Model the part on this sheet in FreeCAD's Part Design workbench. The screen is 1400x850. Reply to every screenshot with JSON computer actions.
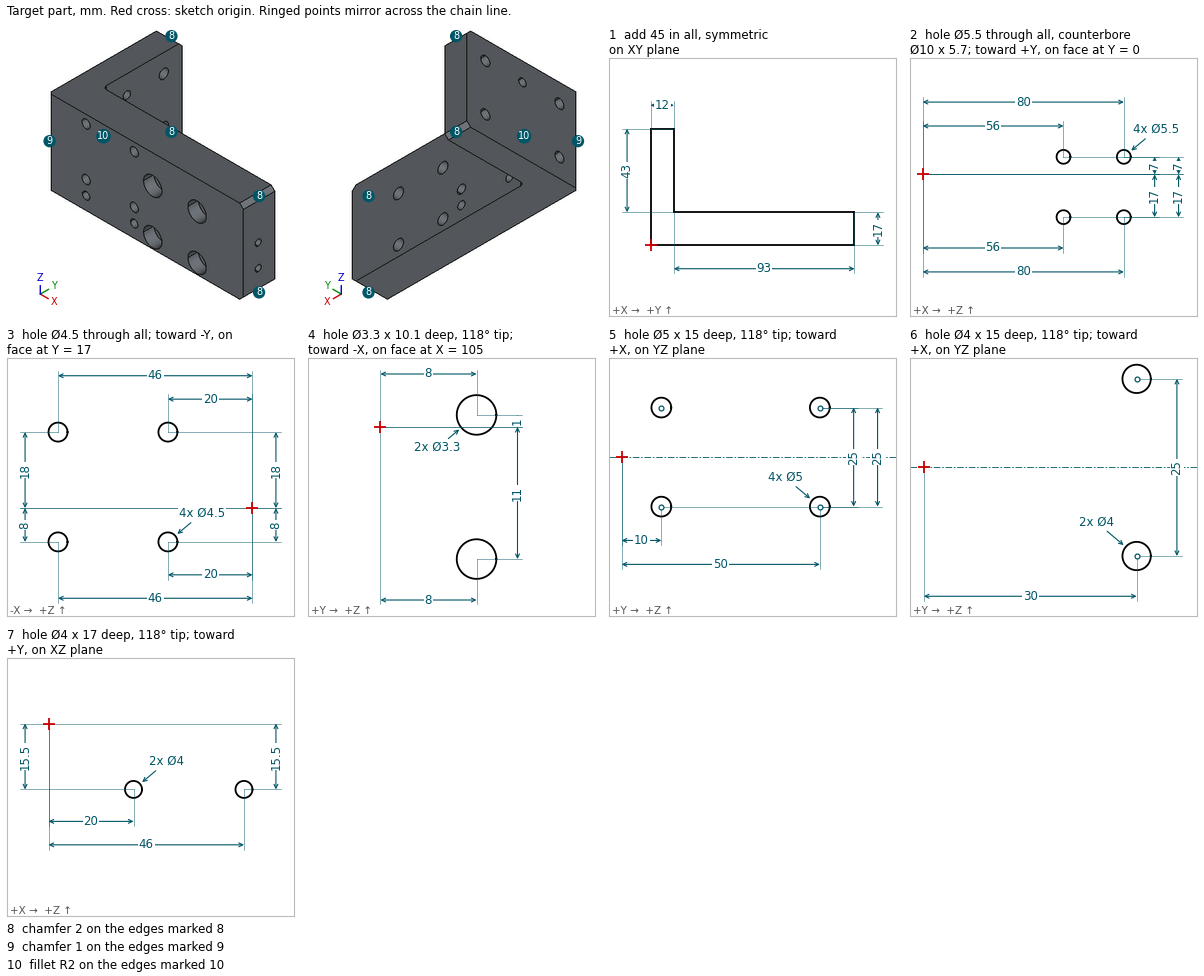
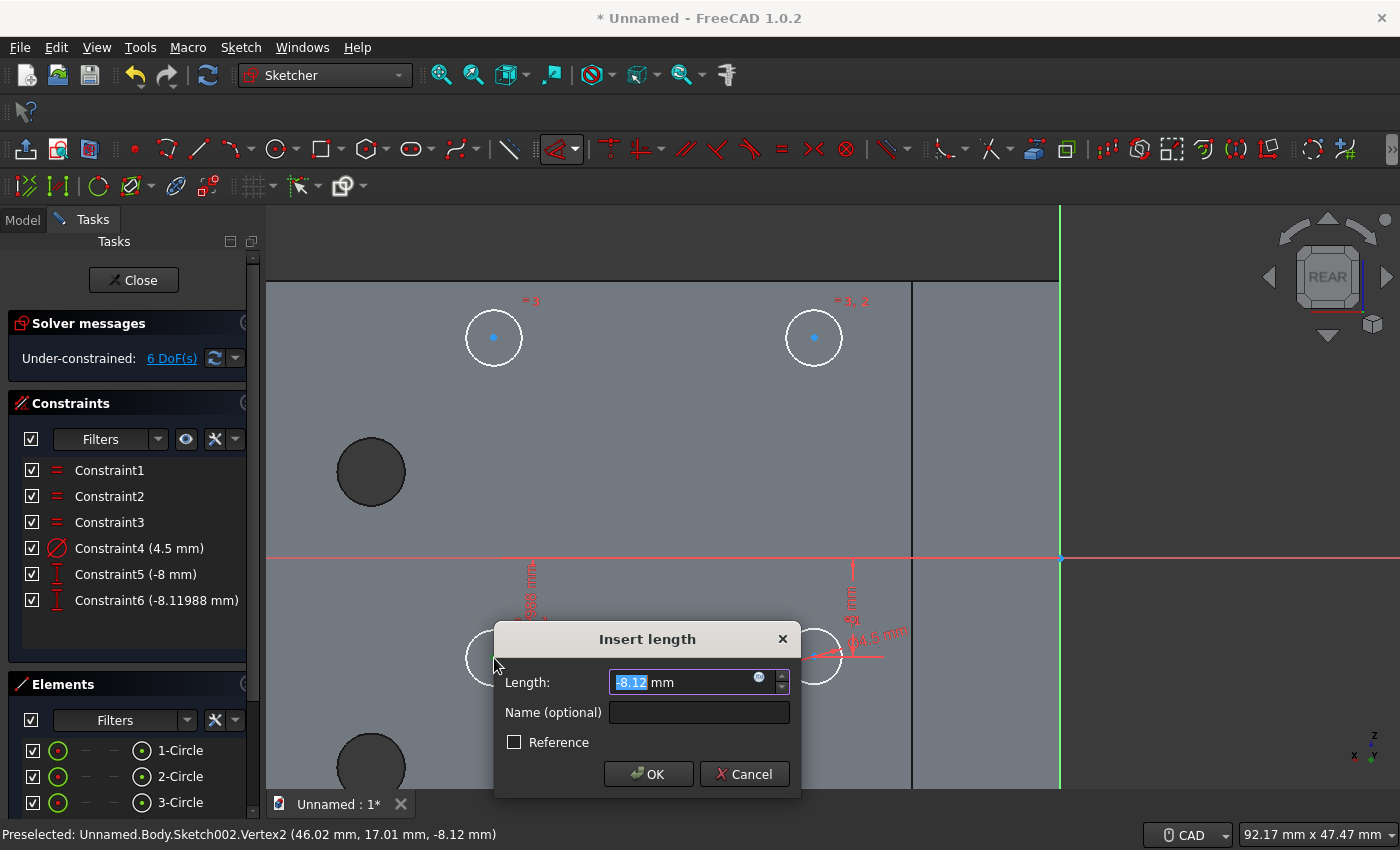
{"action": "type", "text": "-8"}
{"action": "key", "text": "Return"}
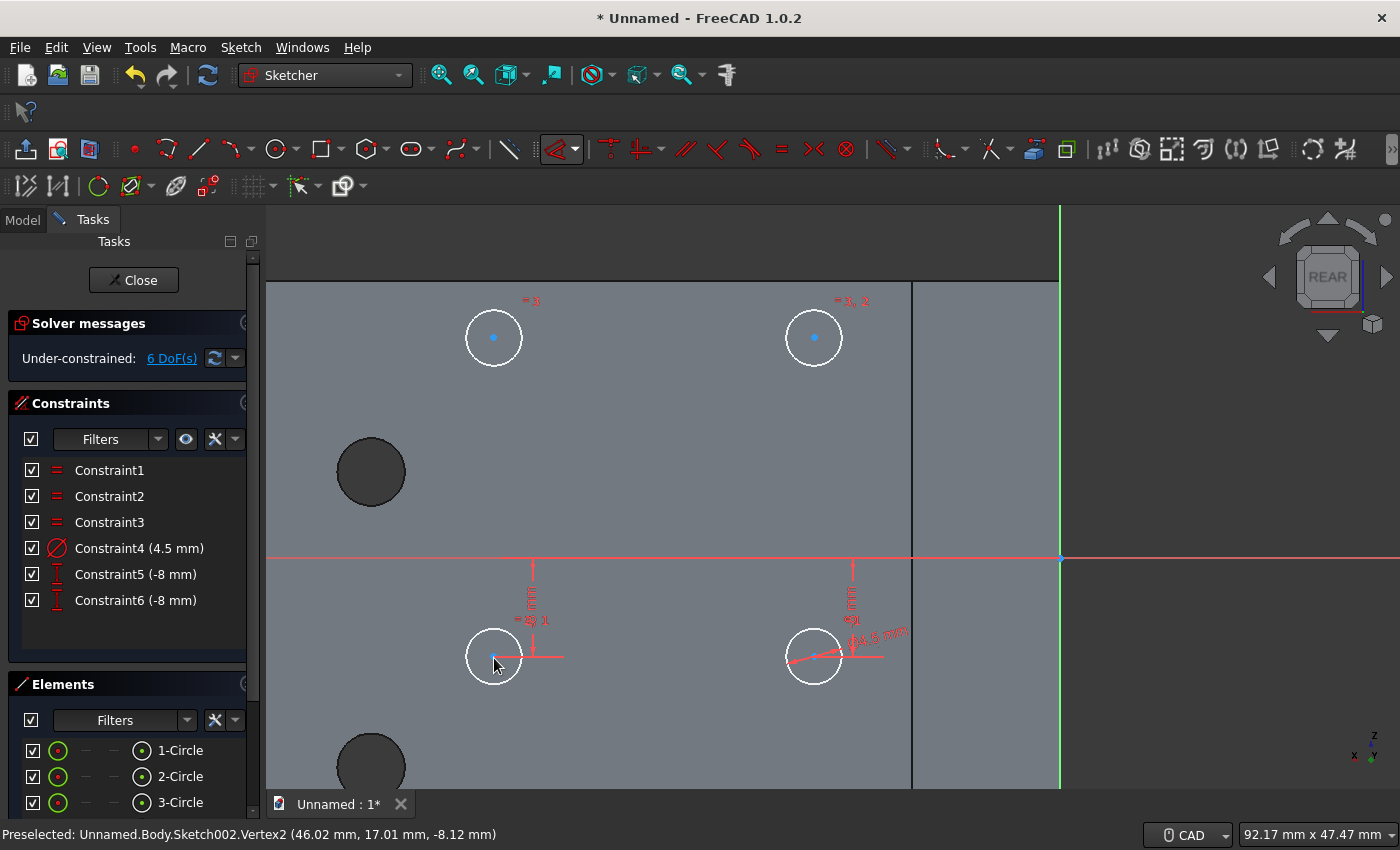
{"action": "left_click", "coordinate": [814, 657]}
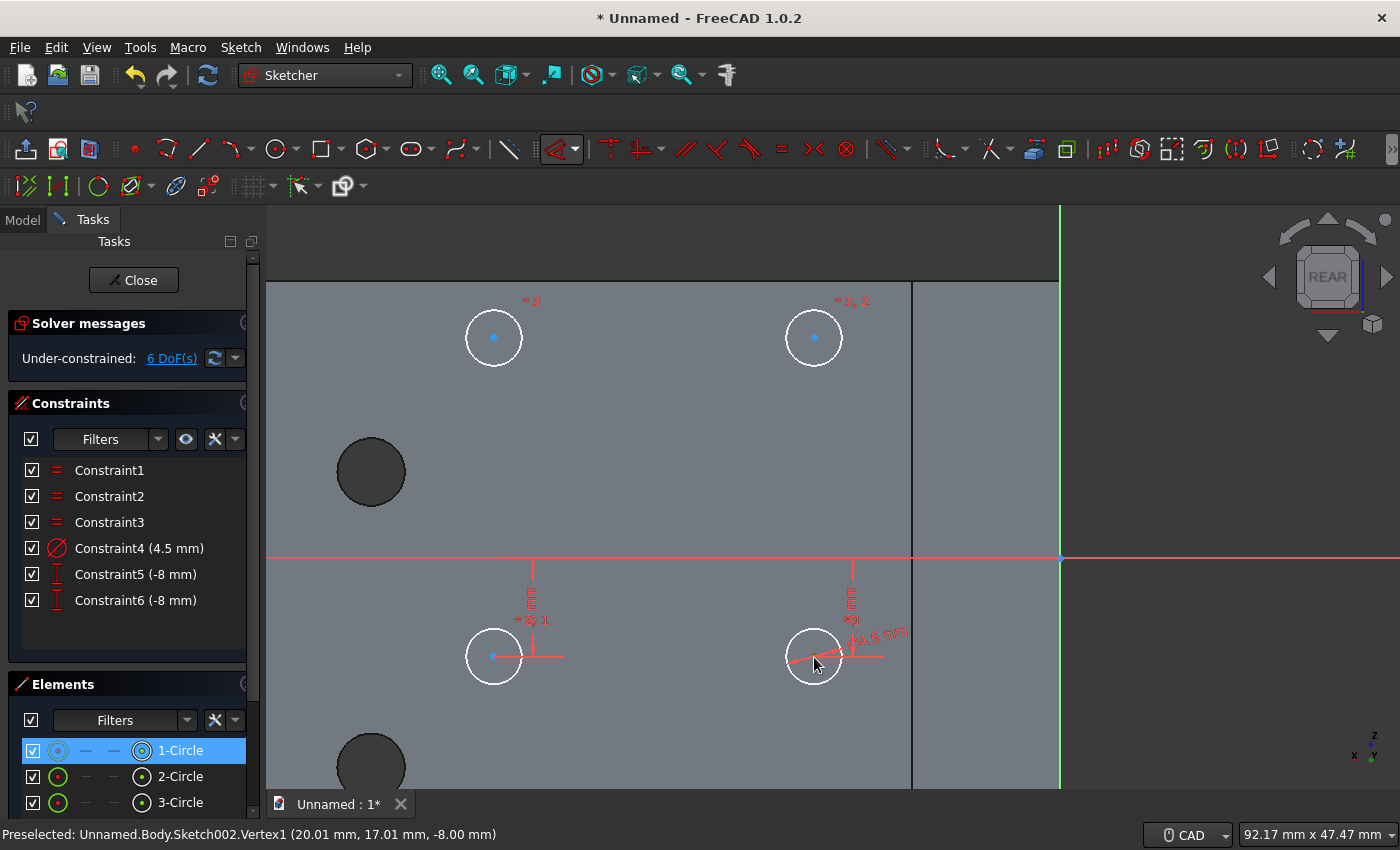
{"action": "key", "text": "l"}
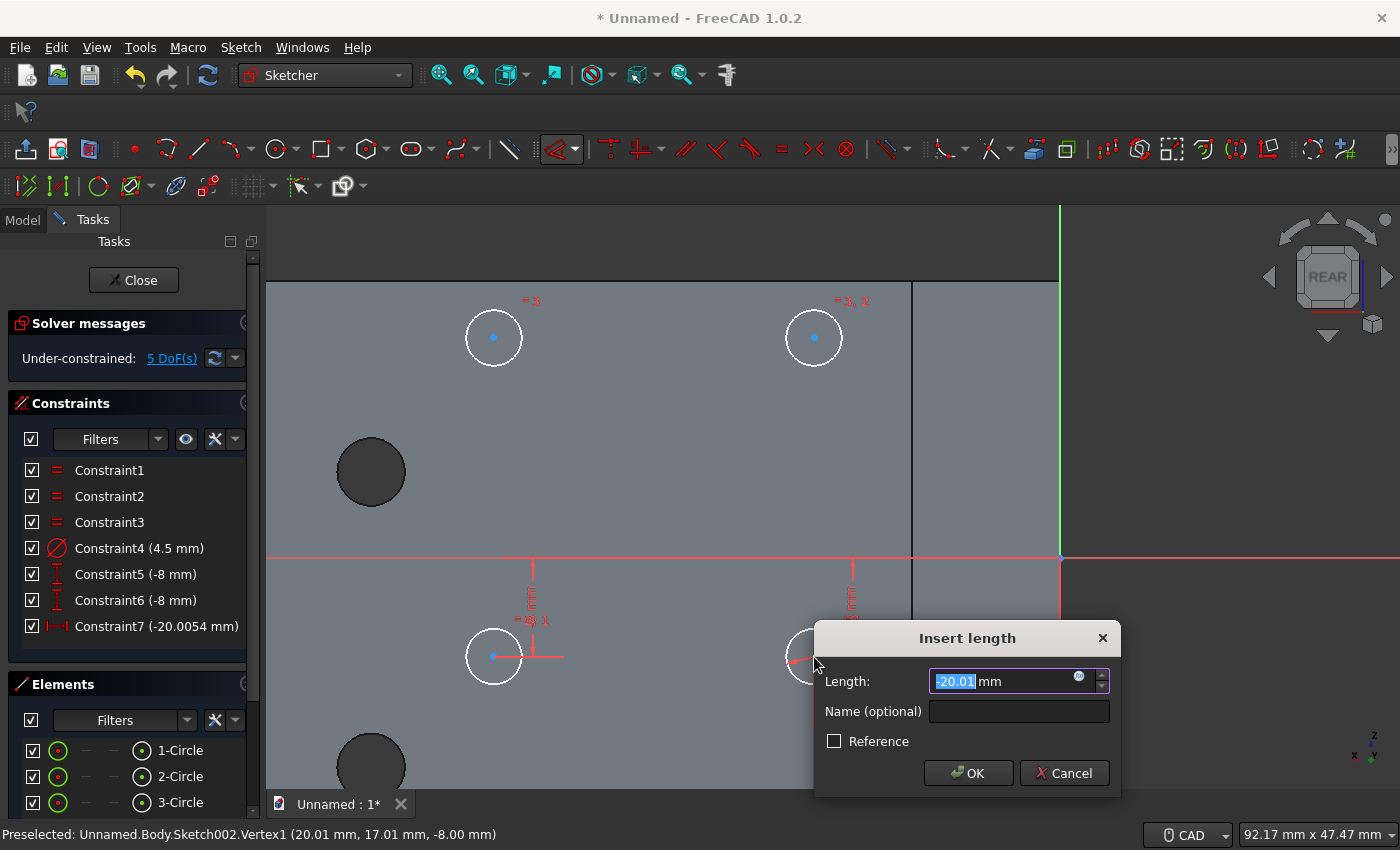
{"action": "type", "text": "-20"}
{"action": "key", "text": "Return"}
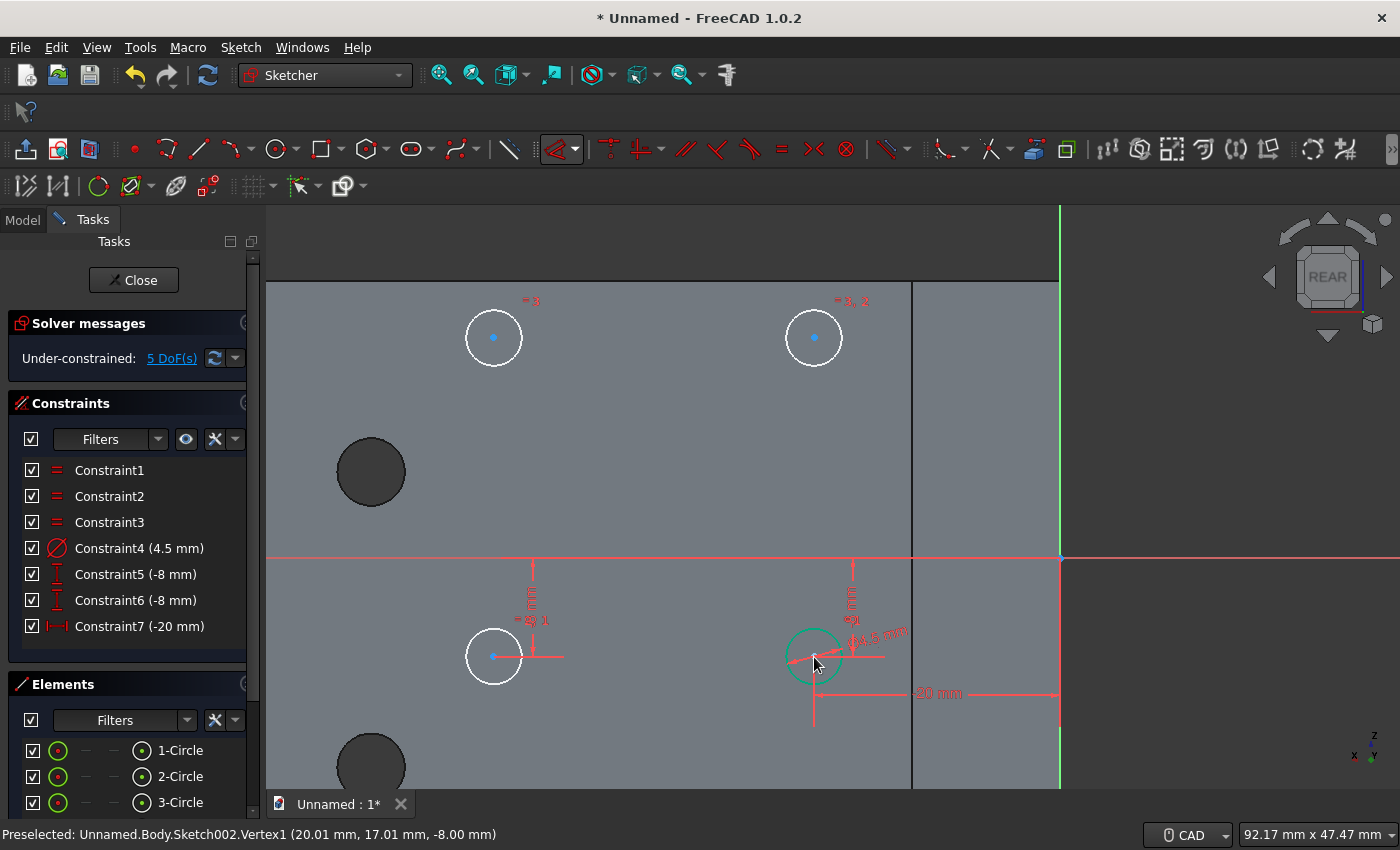
{"action": "left_click", "coordinate": [494, 657]}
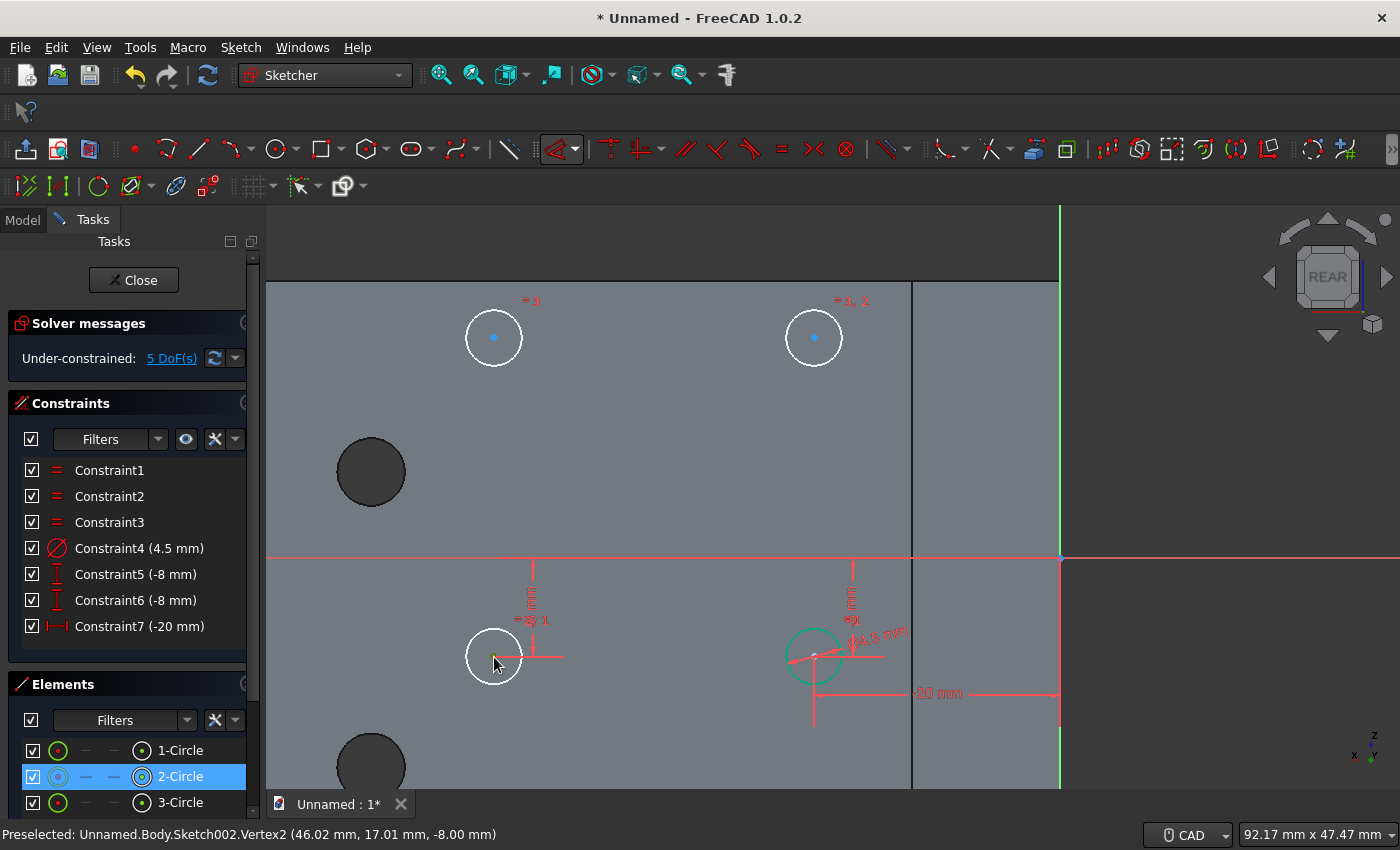
{"action": "key", "text": "l"}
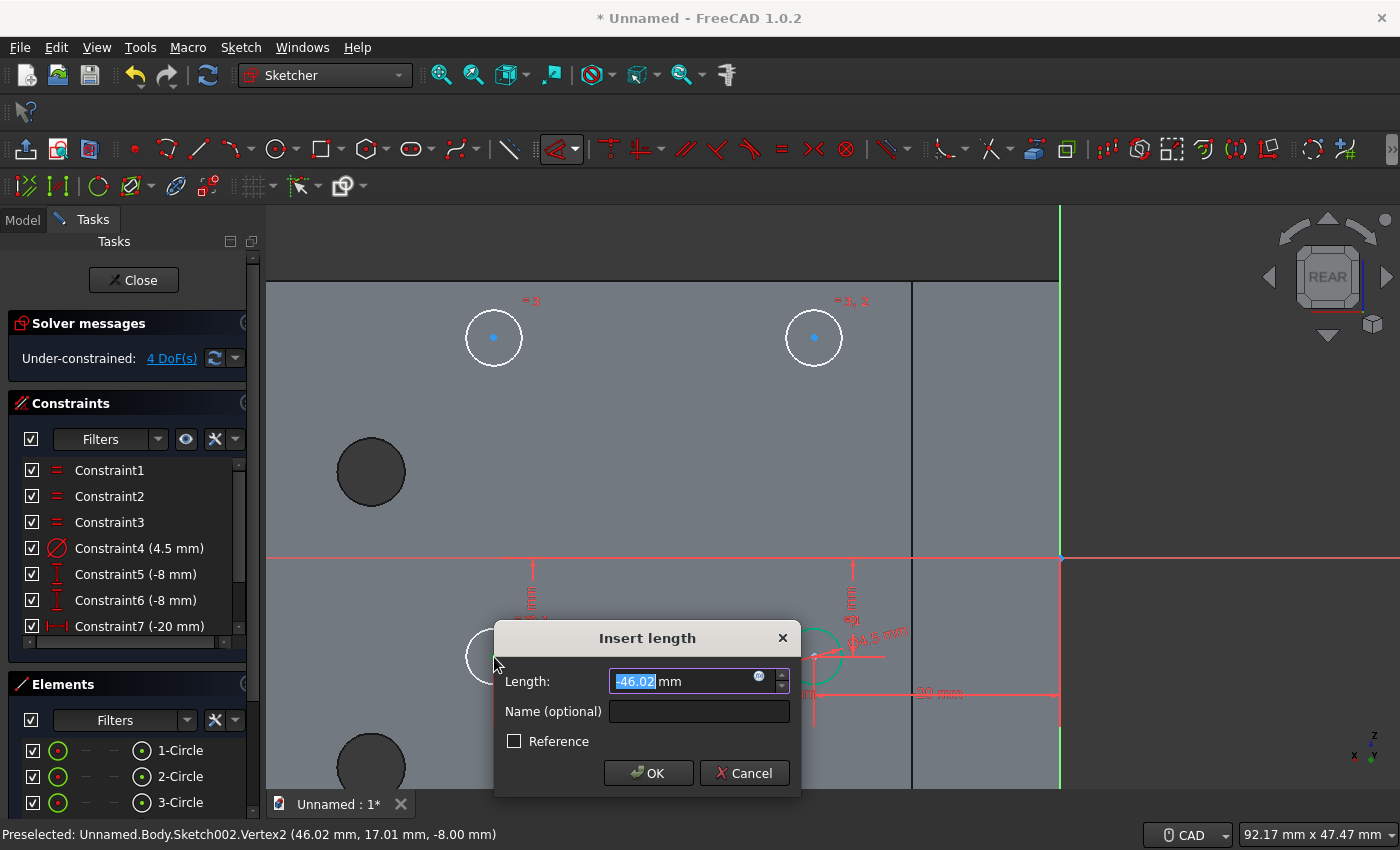
{"action": "type", "text": "-46"}
{"action": "key", "text": "Return"}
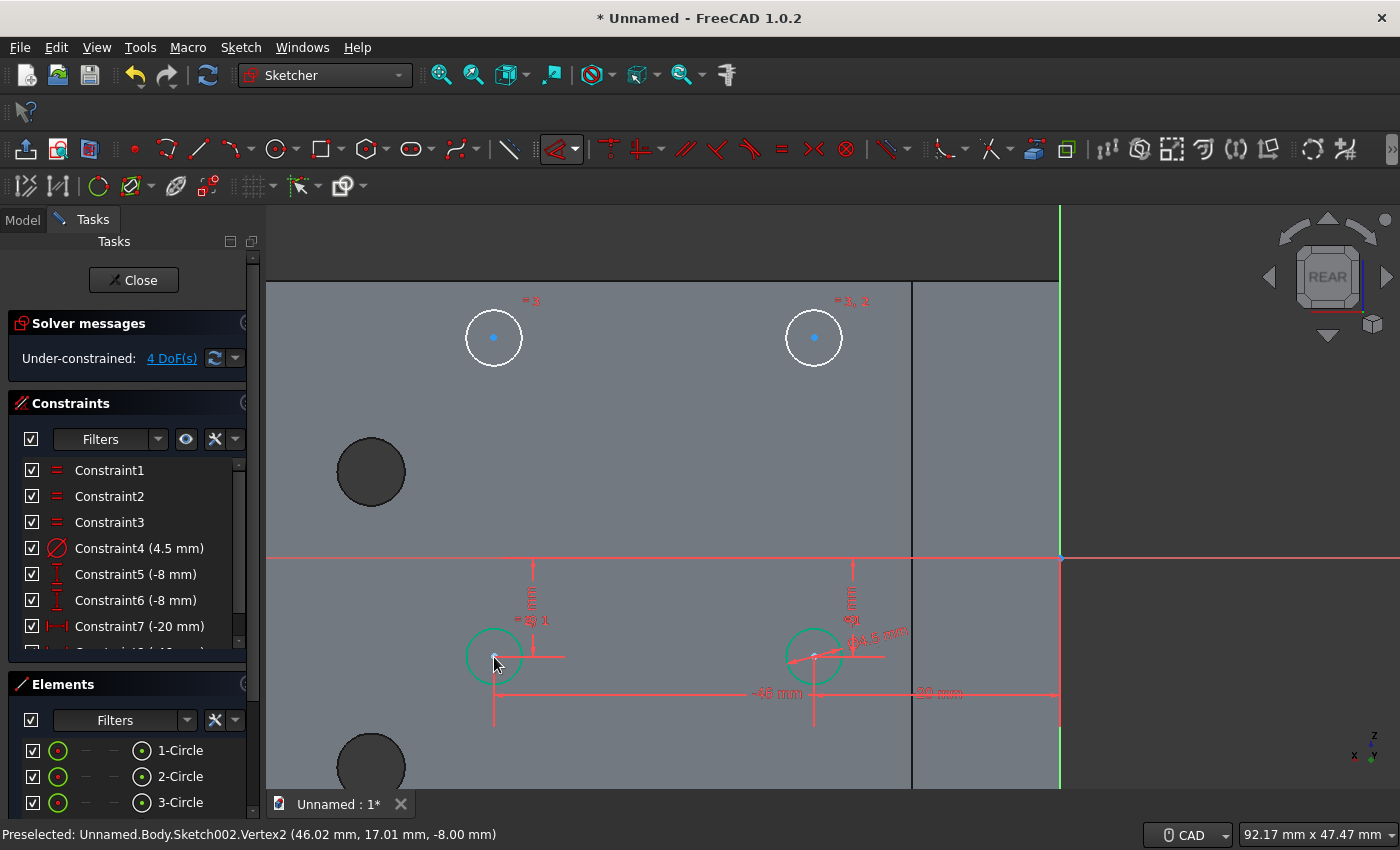
{"action": "left_click", "coordinate": [814, 338]}